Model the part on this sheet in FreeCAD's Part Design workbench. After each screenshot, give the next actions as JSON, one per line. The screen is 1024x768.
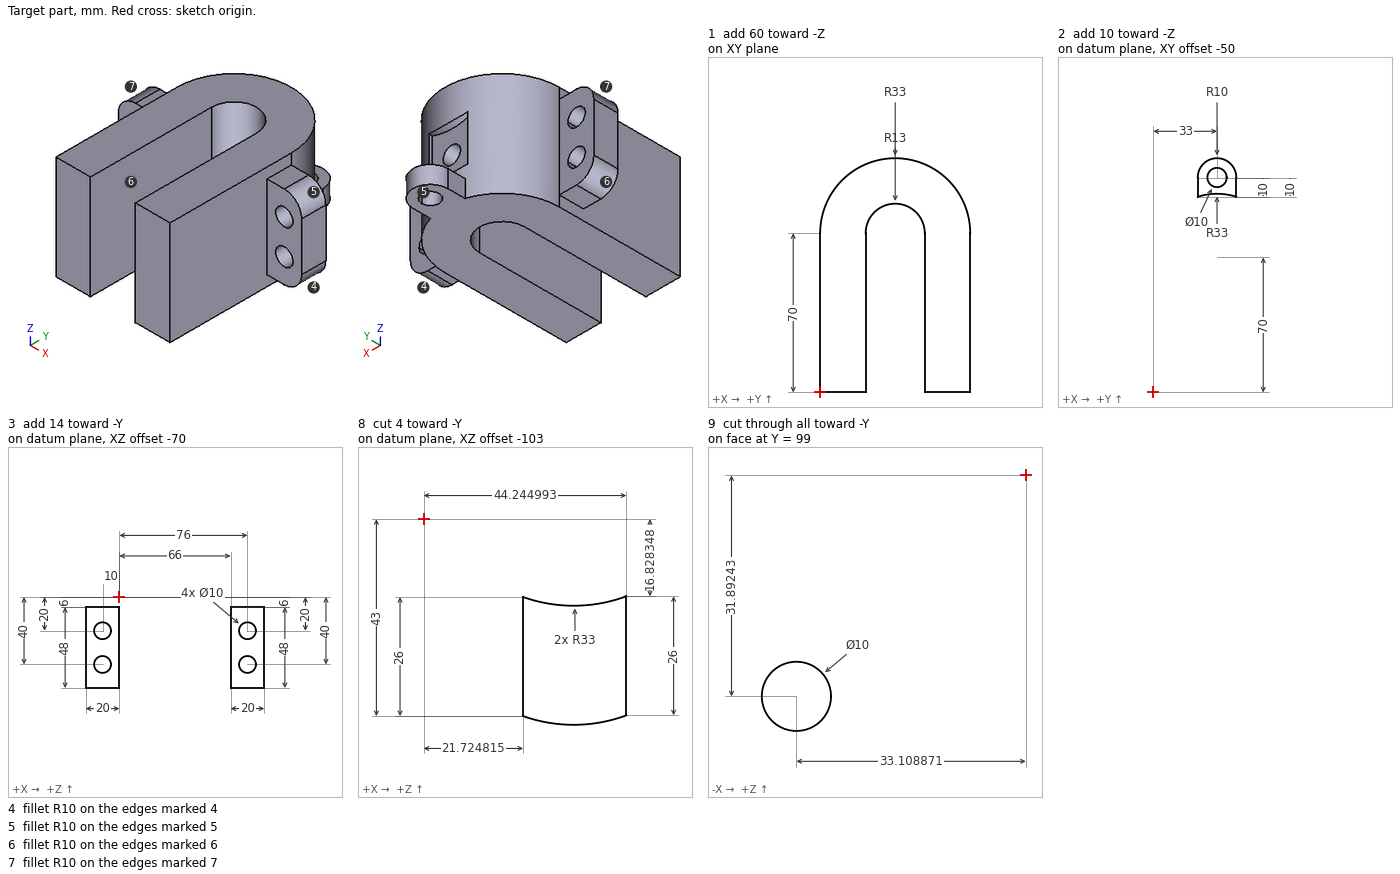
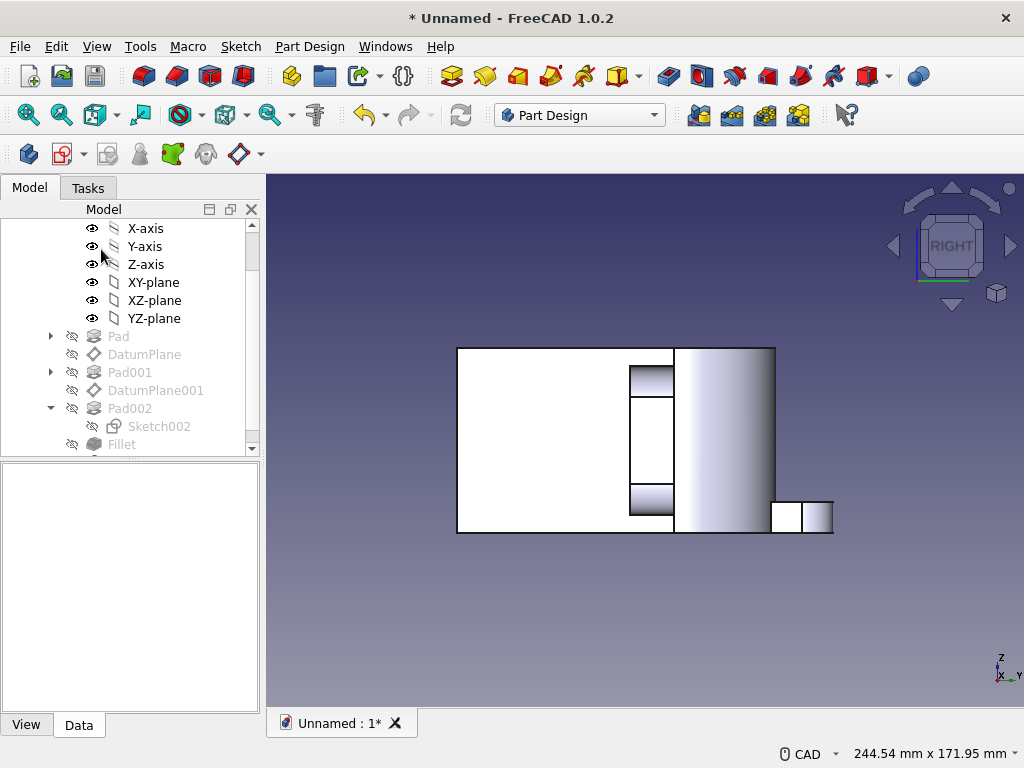
{"action": "key", "text": "0"}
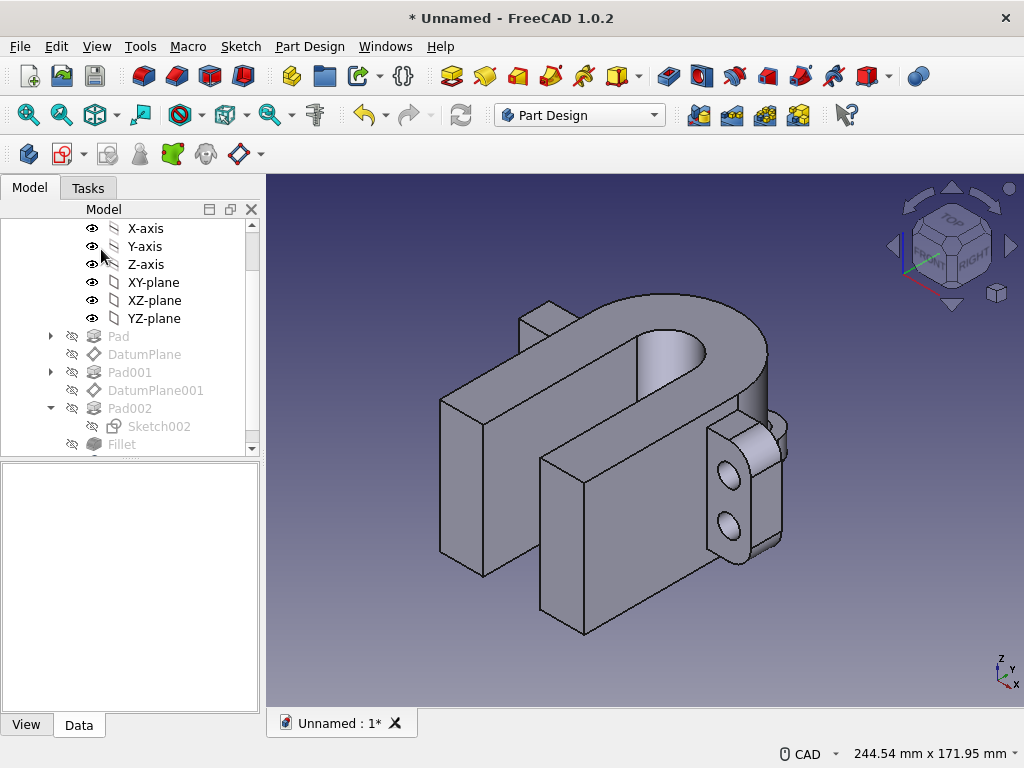
{"action": "key", "text": "2"}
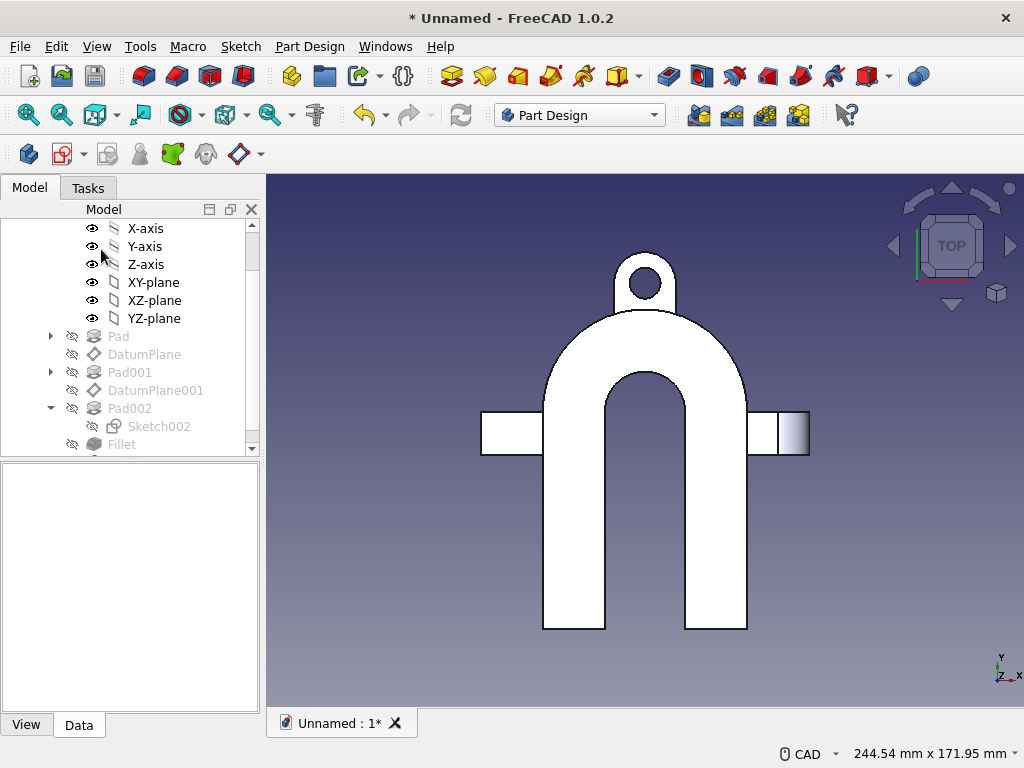
{"action": "key", "text": "1"}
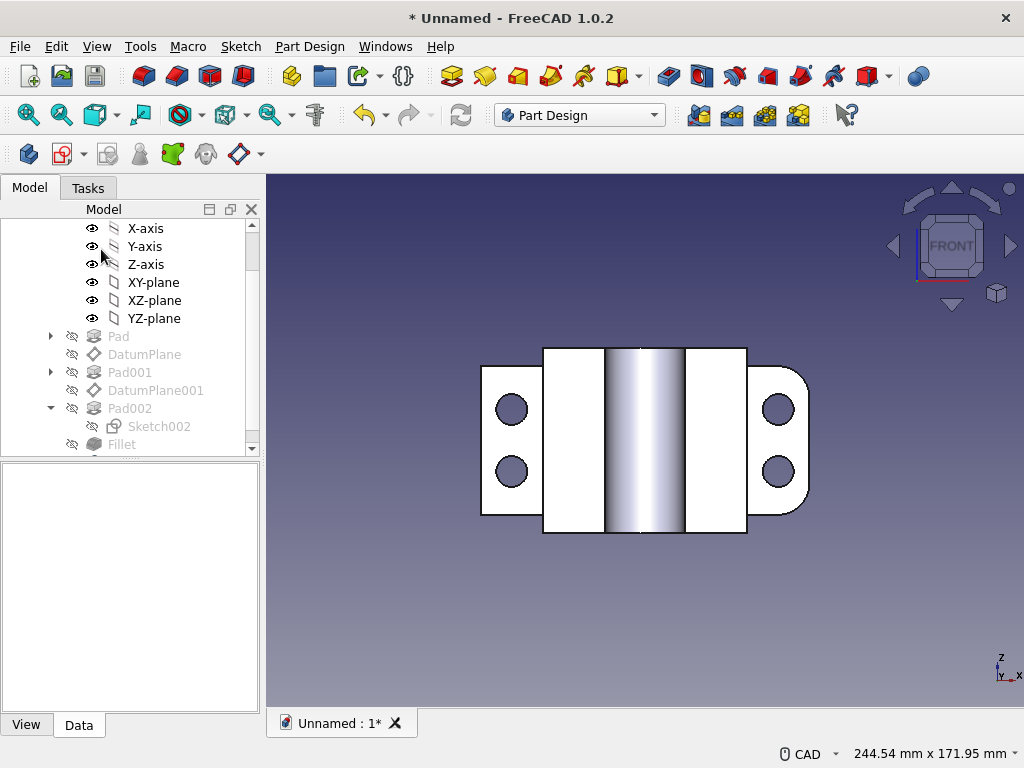
{"action": "left_click", "coordinate": [29, 116]}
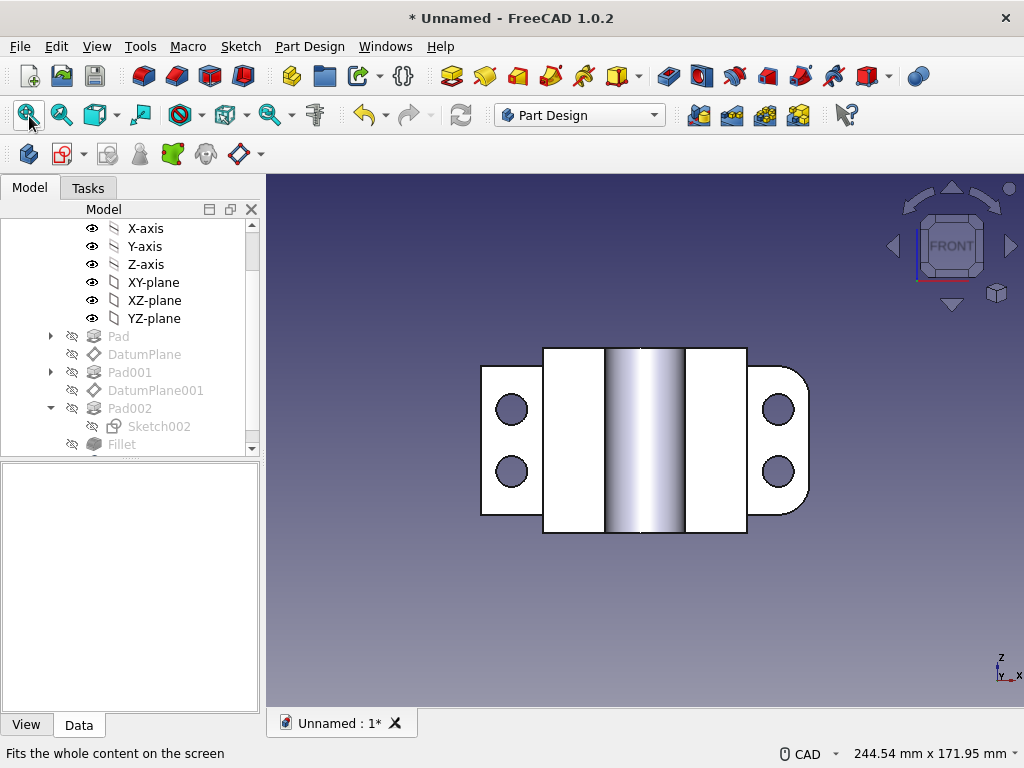
{"action": "key", "text": "3"}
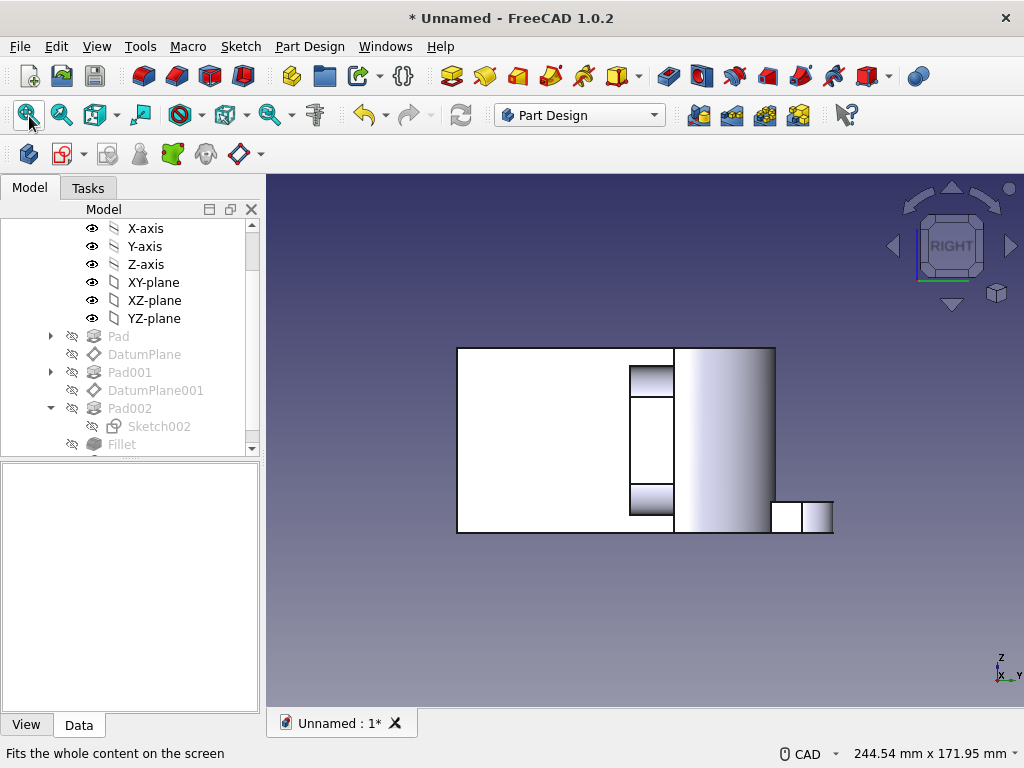
{"action": "key", "text": "5"}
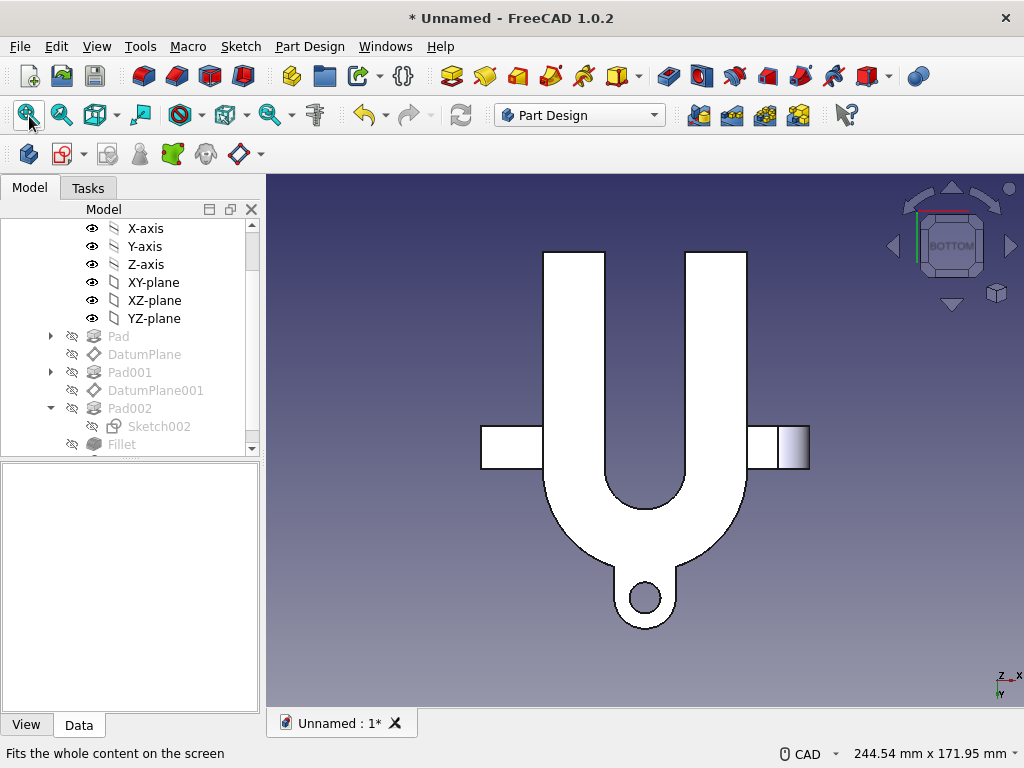
{"action": "left_click", "coordinate": [481, 447]}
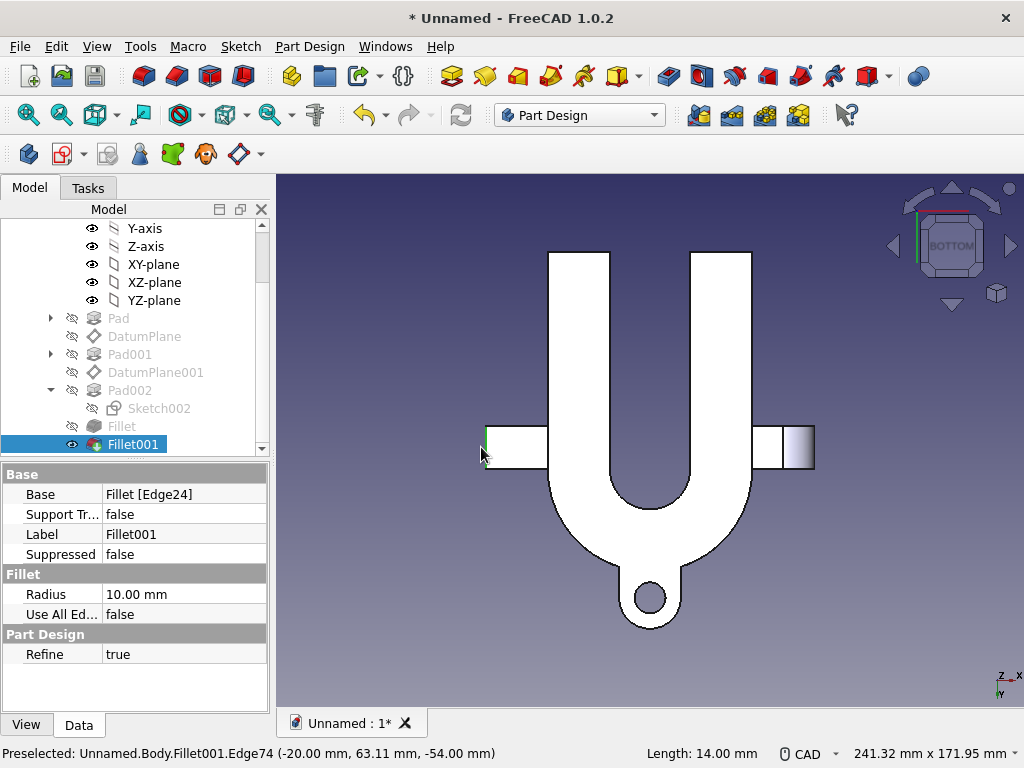
{"action": "left_click", "coordinate": [144, 76]}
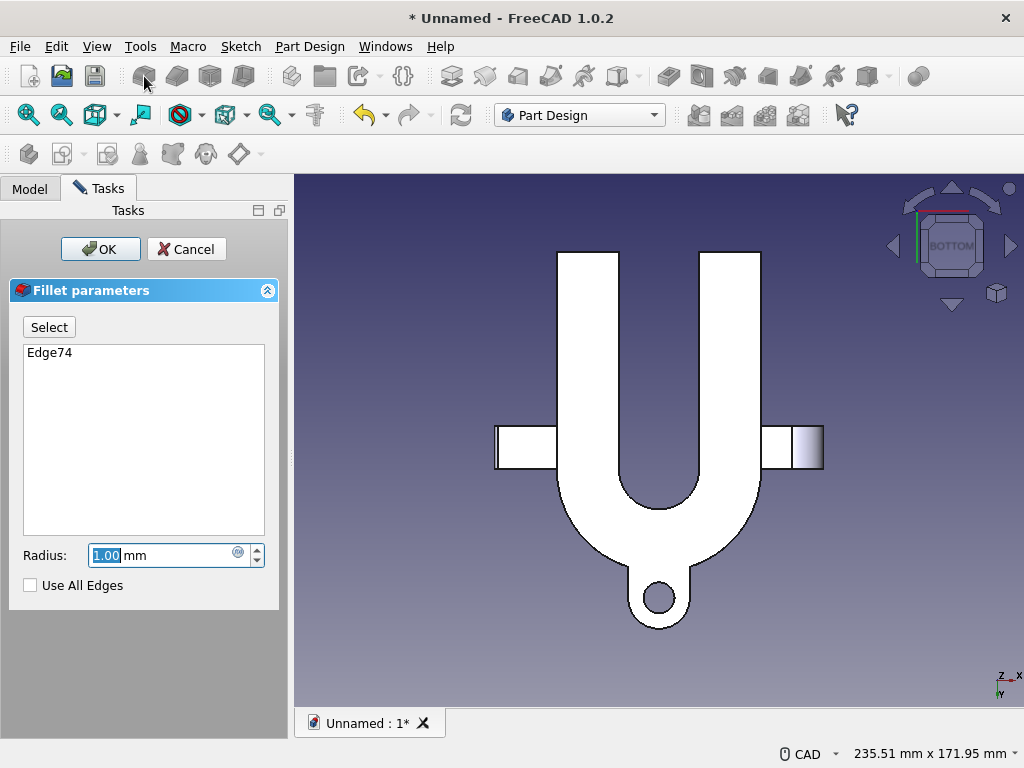
{"action": "type", "text": "10"}
{"action": "key", "text": "Tab"}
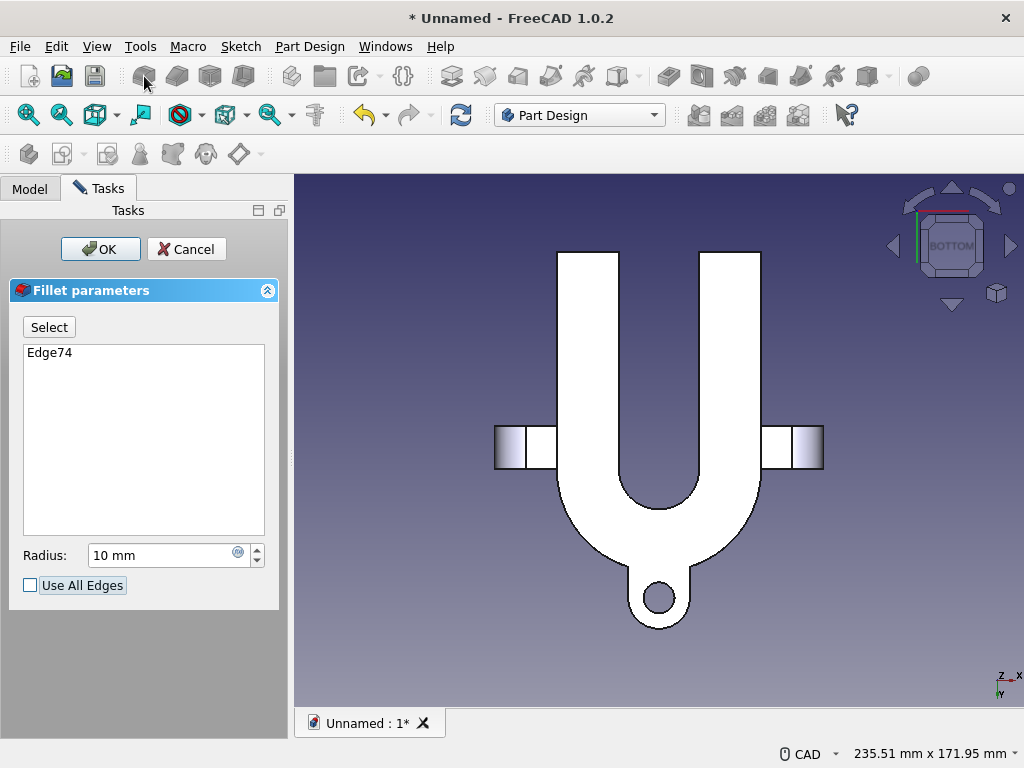
{"action": "left_click", "coordinate": [101, 249]}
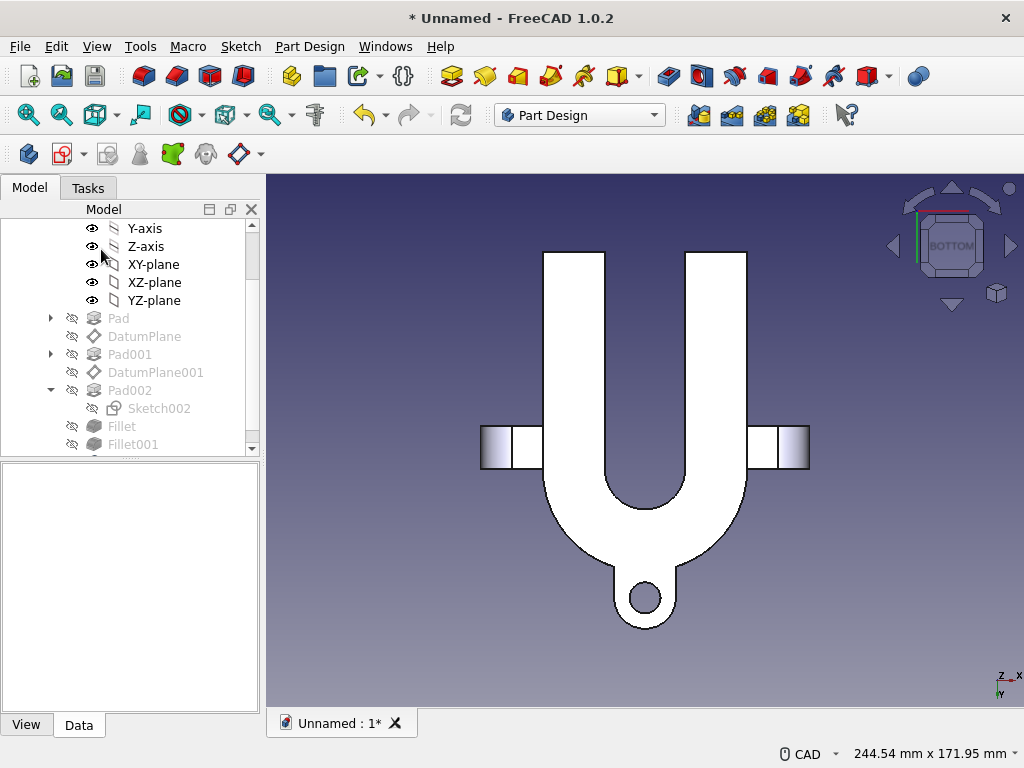
{"action": "key", "text": "0"}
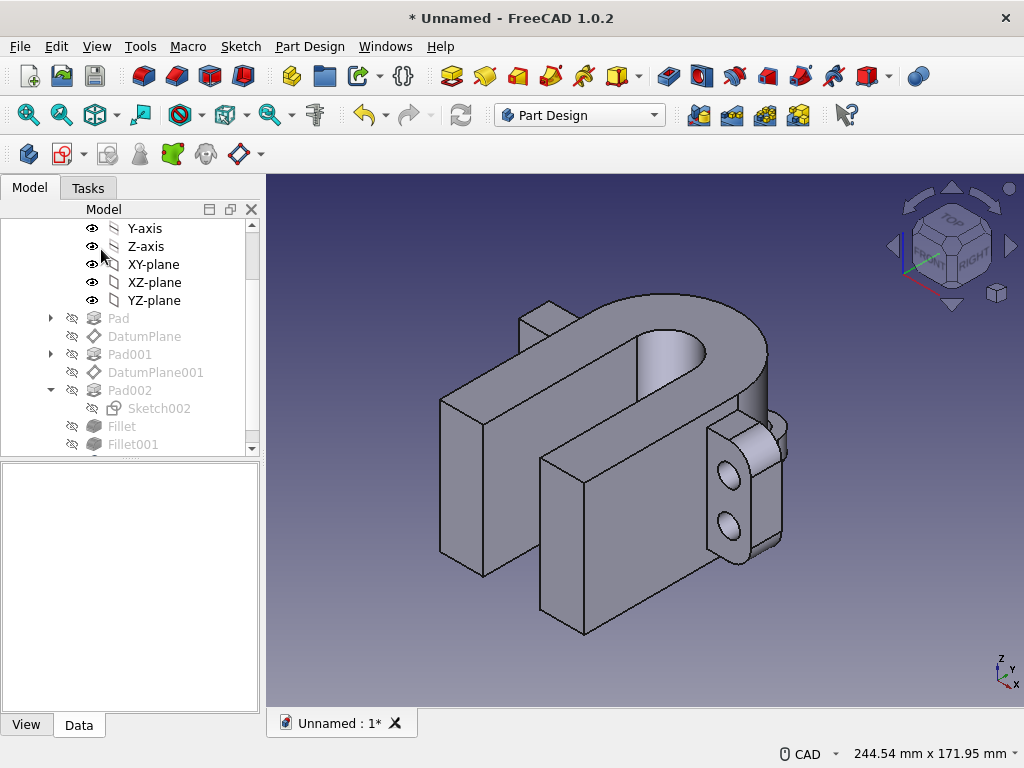
{"action": "key", "text": "2"}